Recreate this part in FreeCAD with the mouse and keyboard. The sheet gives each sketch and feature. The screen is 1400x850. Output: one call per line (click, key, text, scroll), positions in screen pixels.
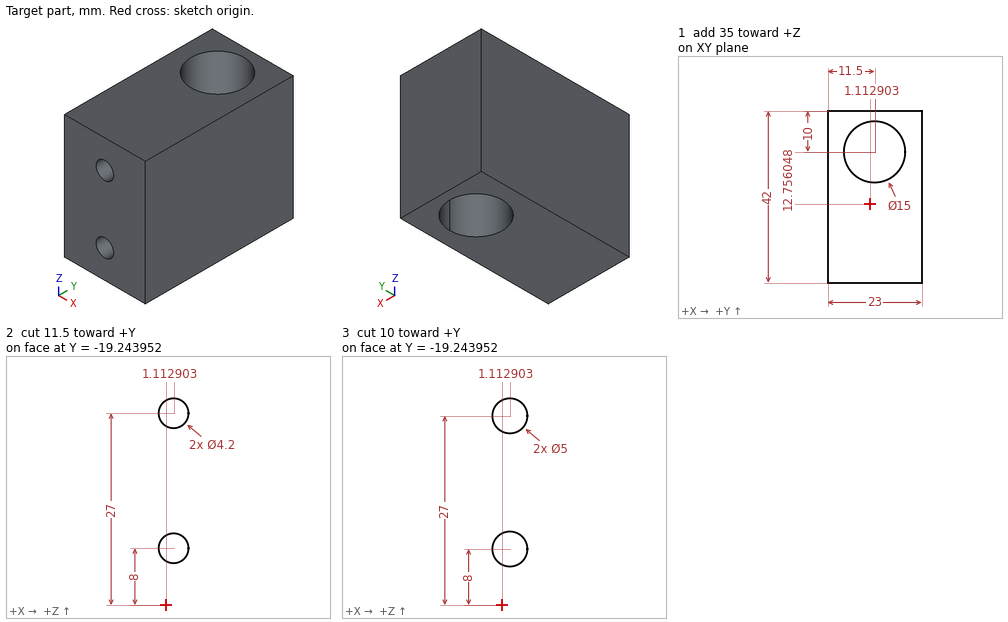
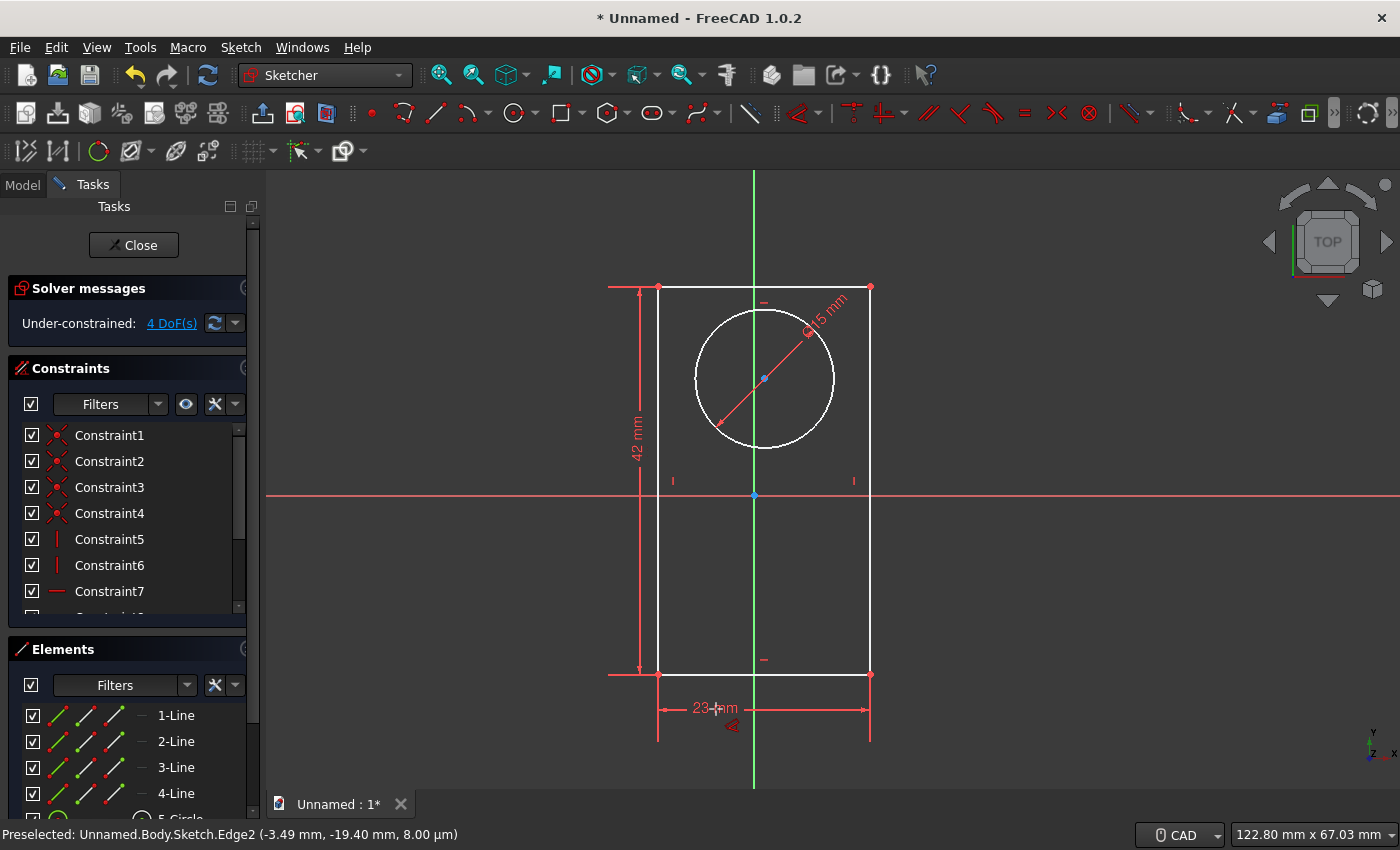
click(658, 287)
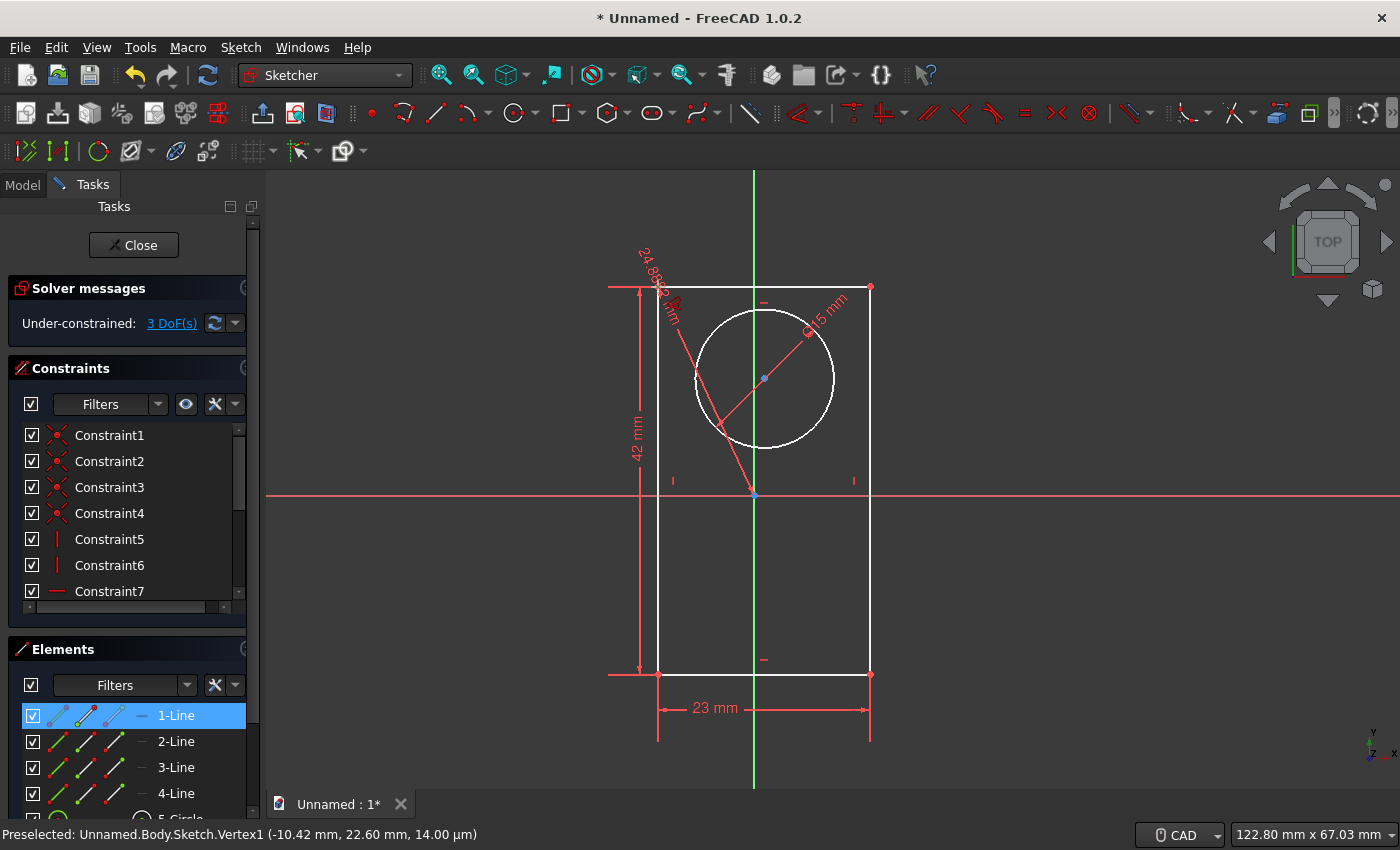
click(765, 379)
click(624, 333)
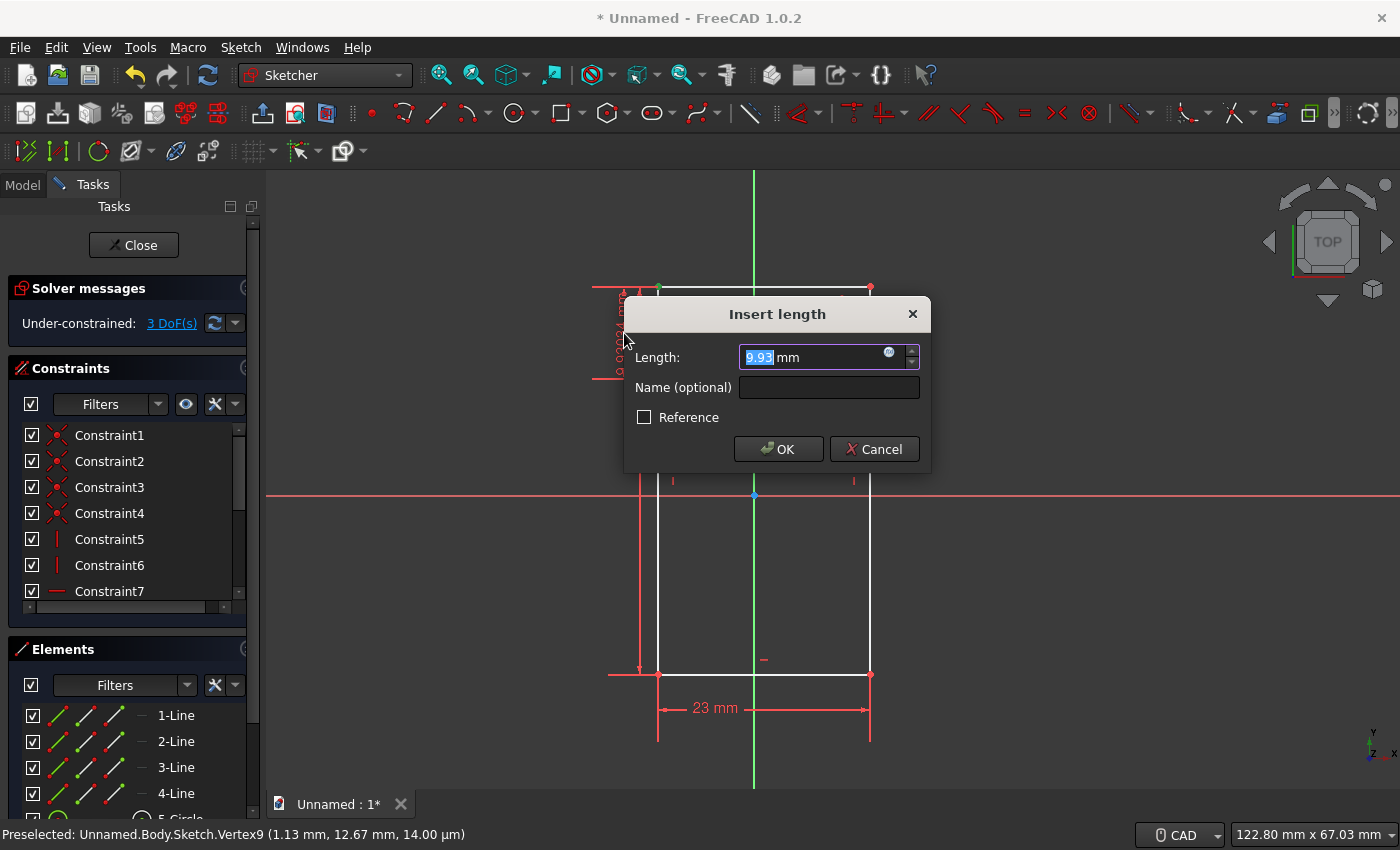
text(10)
key(Return)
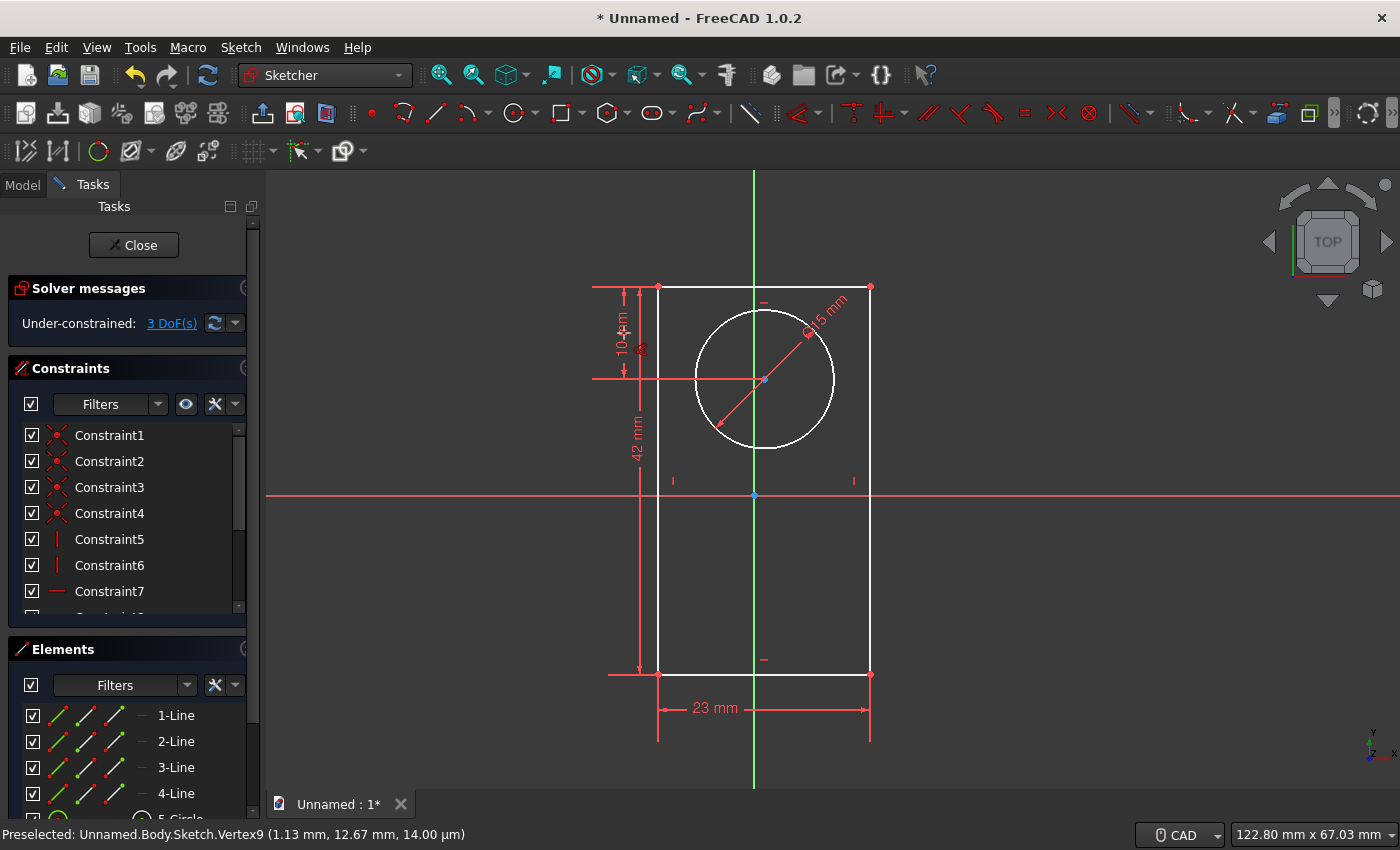
click(658, 287)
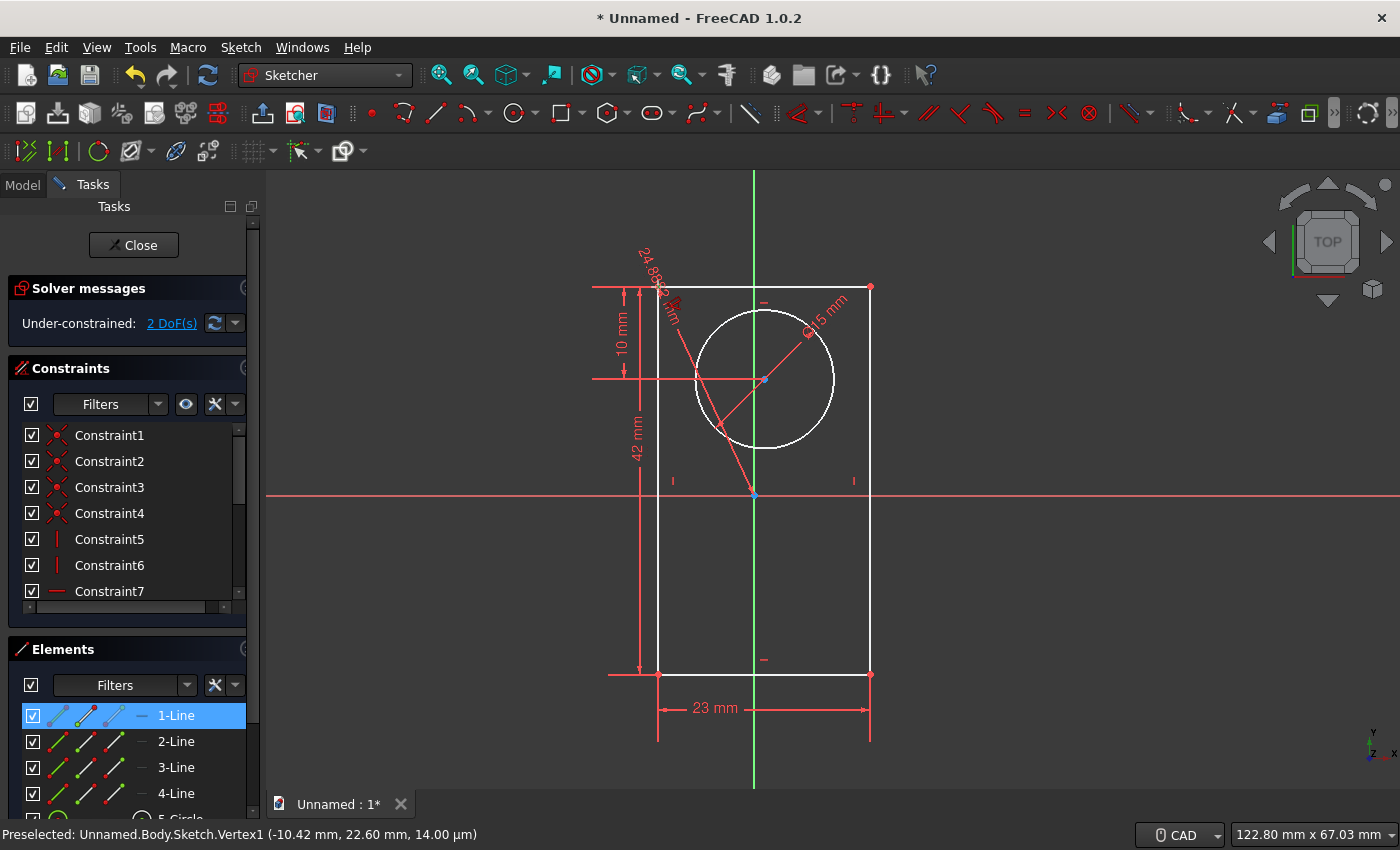
click(765, 379)
click(711, 253)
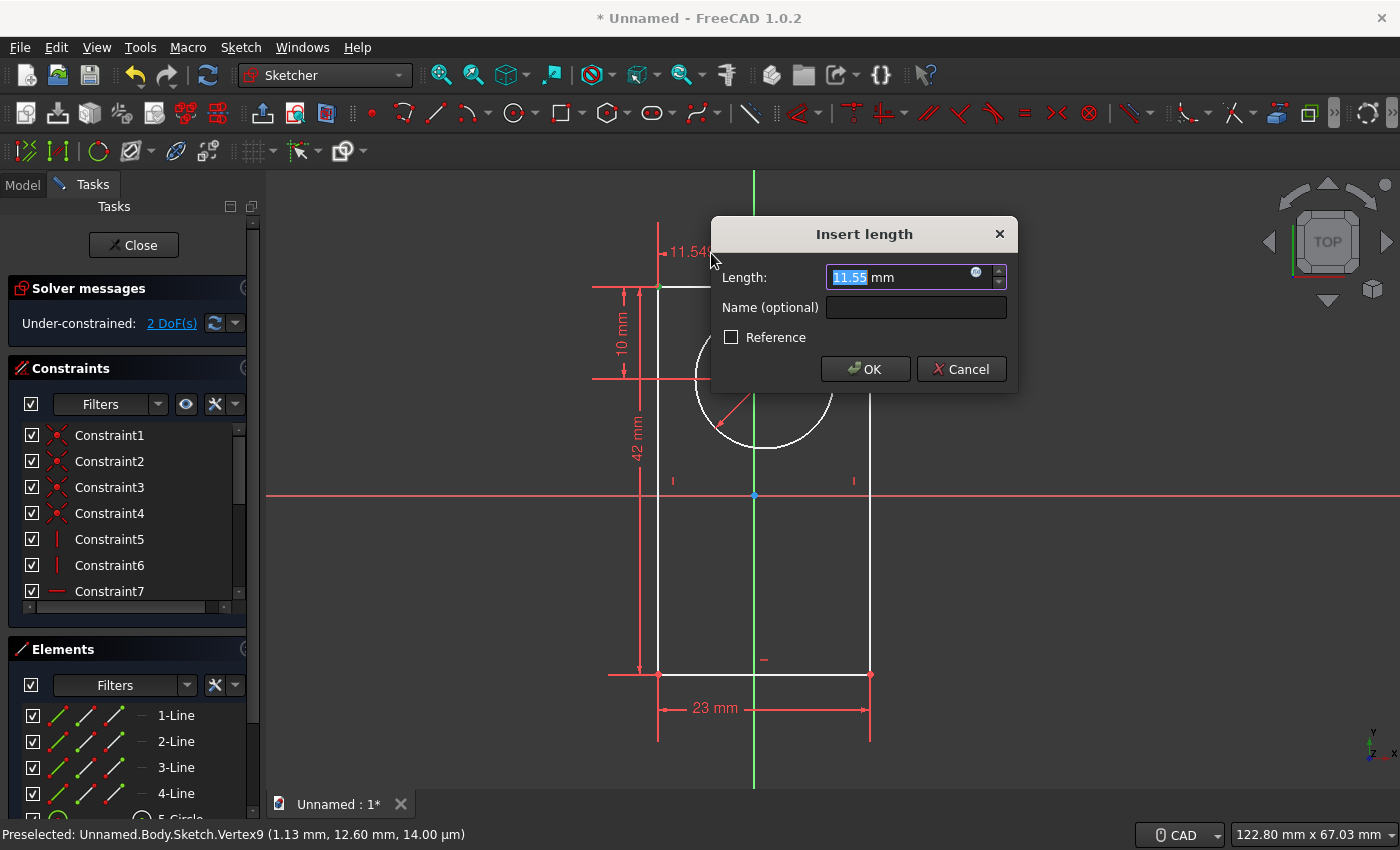
text(11.5)
key(Return)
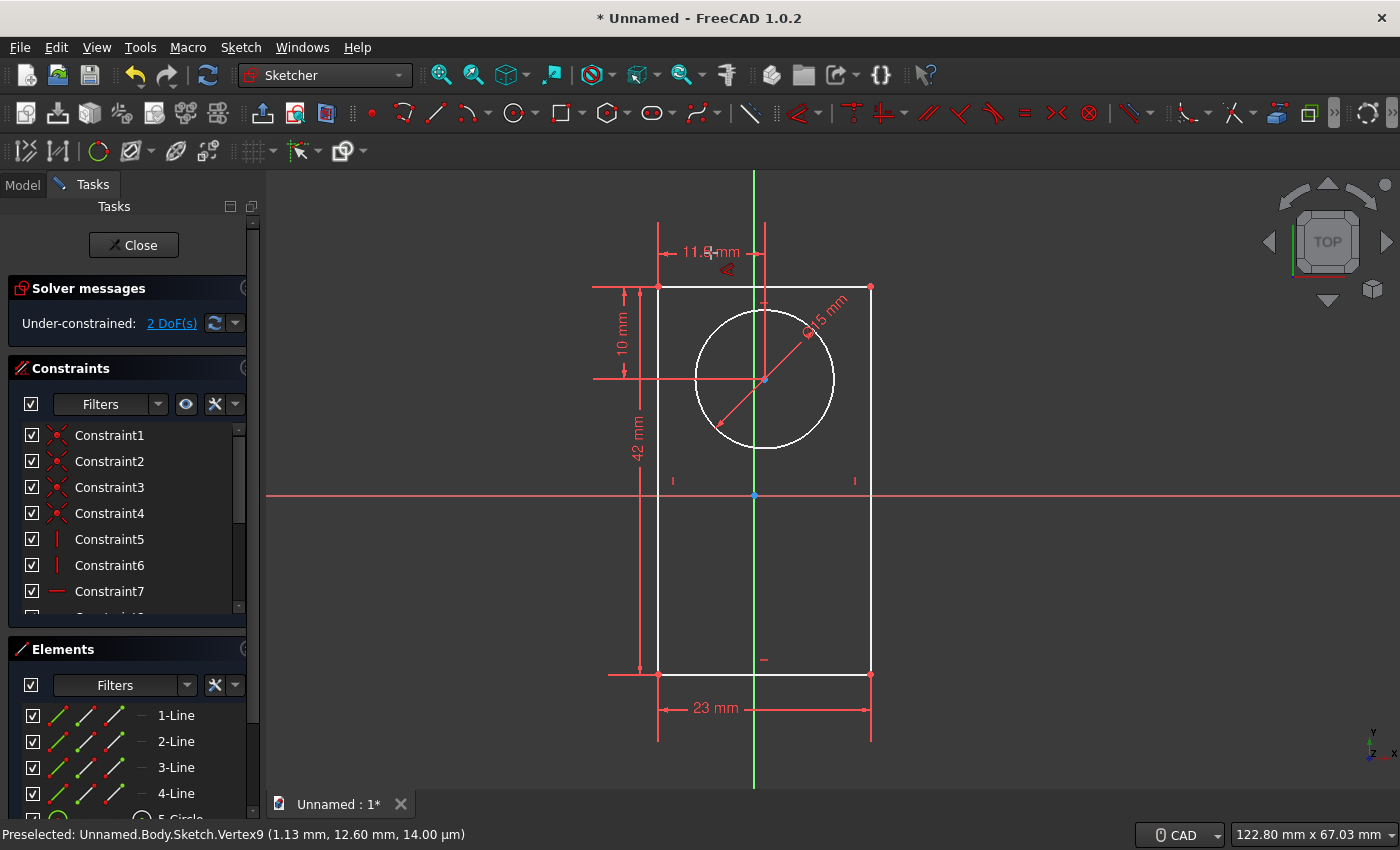
scroll(765, 379, up, 7)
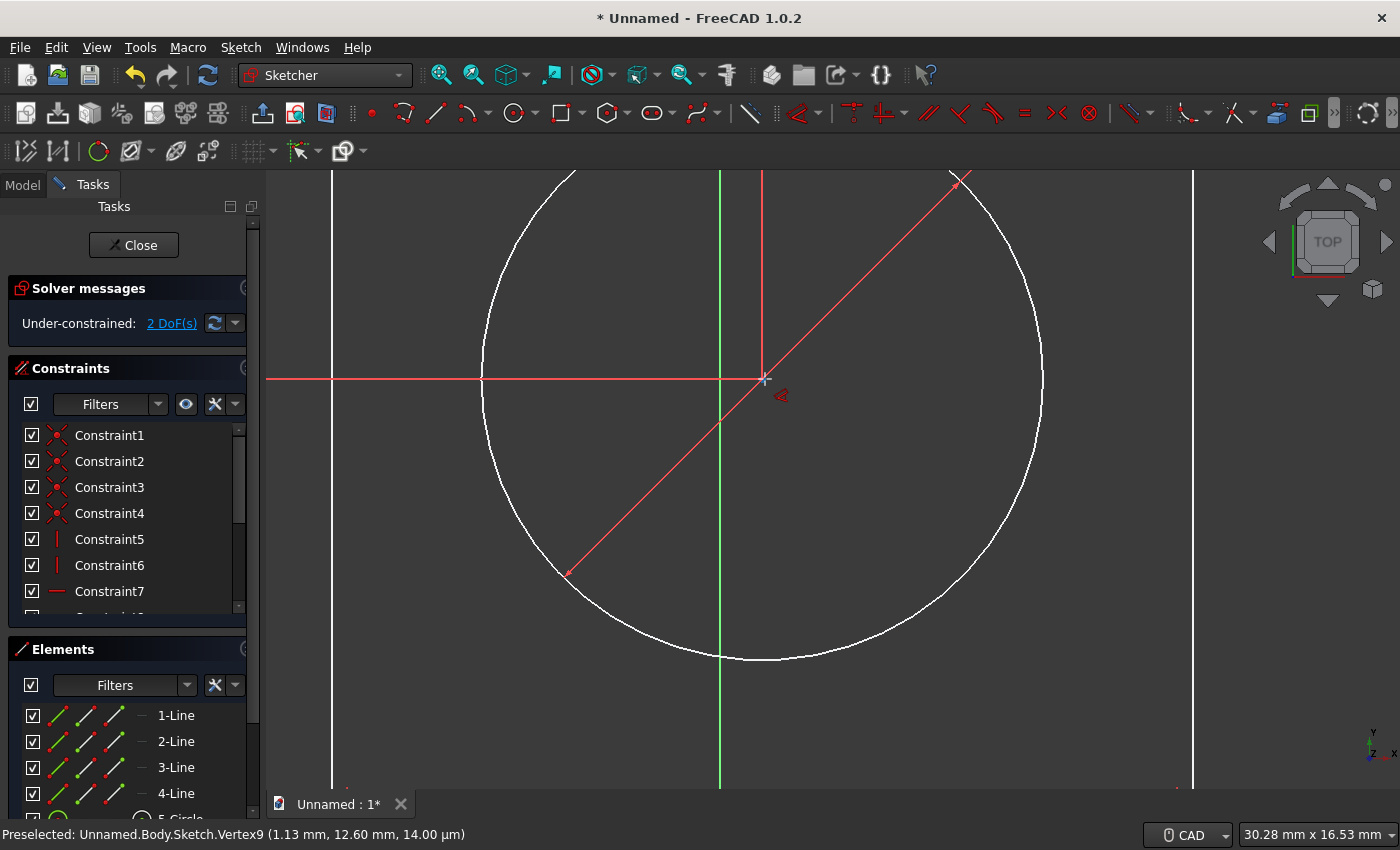
click(762, 379)
click(741, 345)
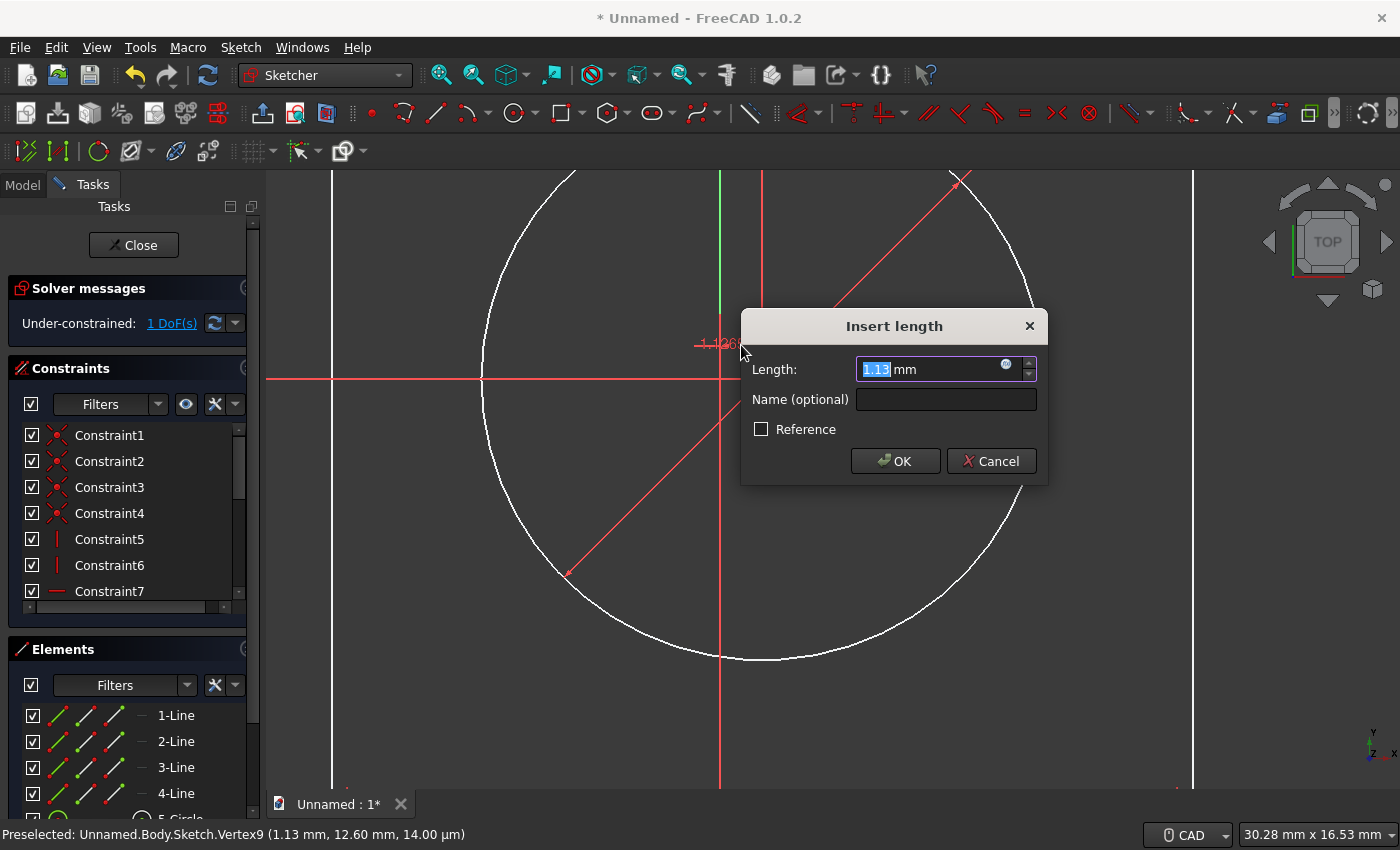
text(1.112903)
key(Return)